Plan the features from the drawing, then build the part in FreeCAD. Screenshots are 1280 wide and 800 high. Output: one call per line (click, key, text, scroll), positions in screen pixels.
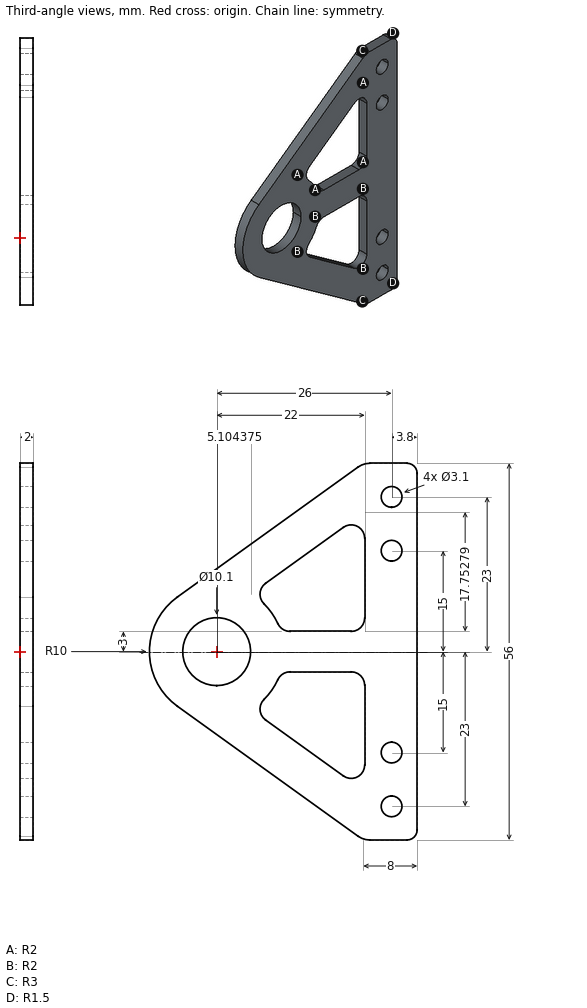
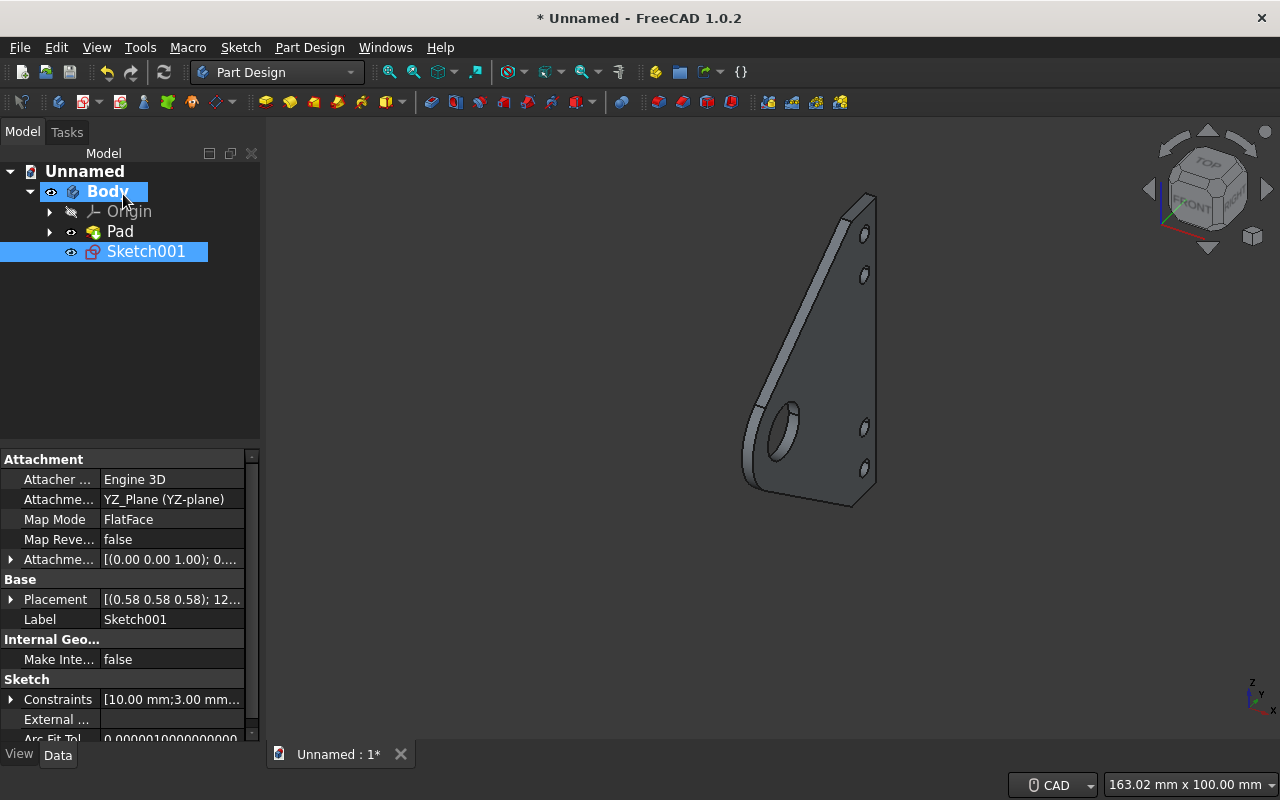
click(432, 102)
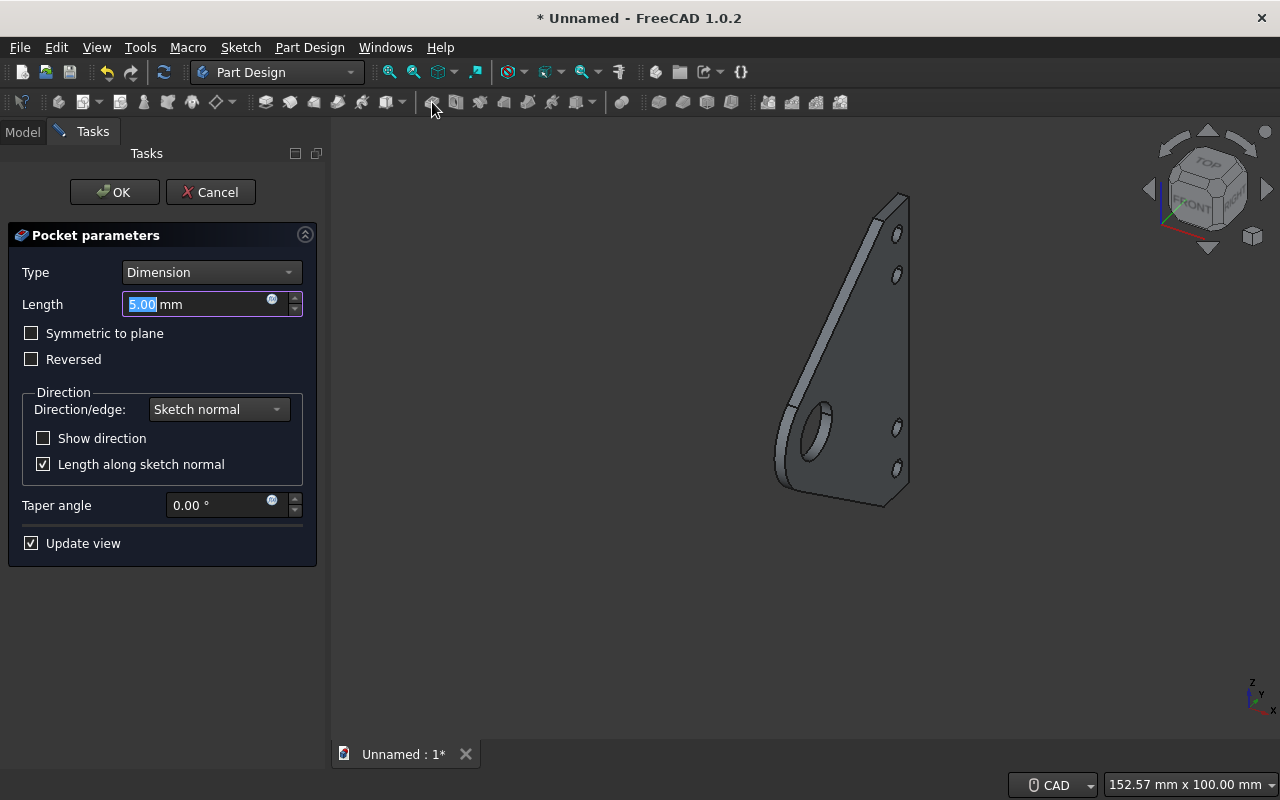
click(212, 272)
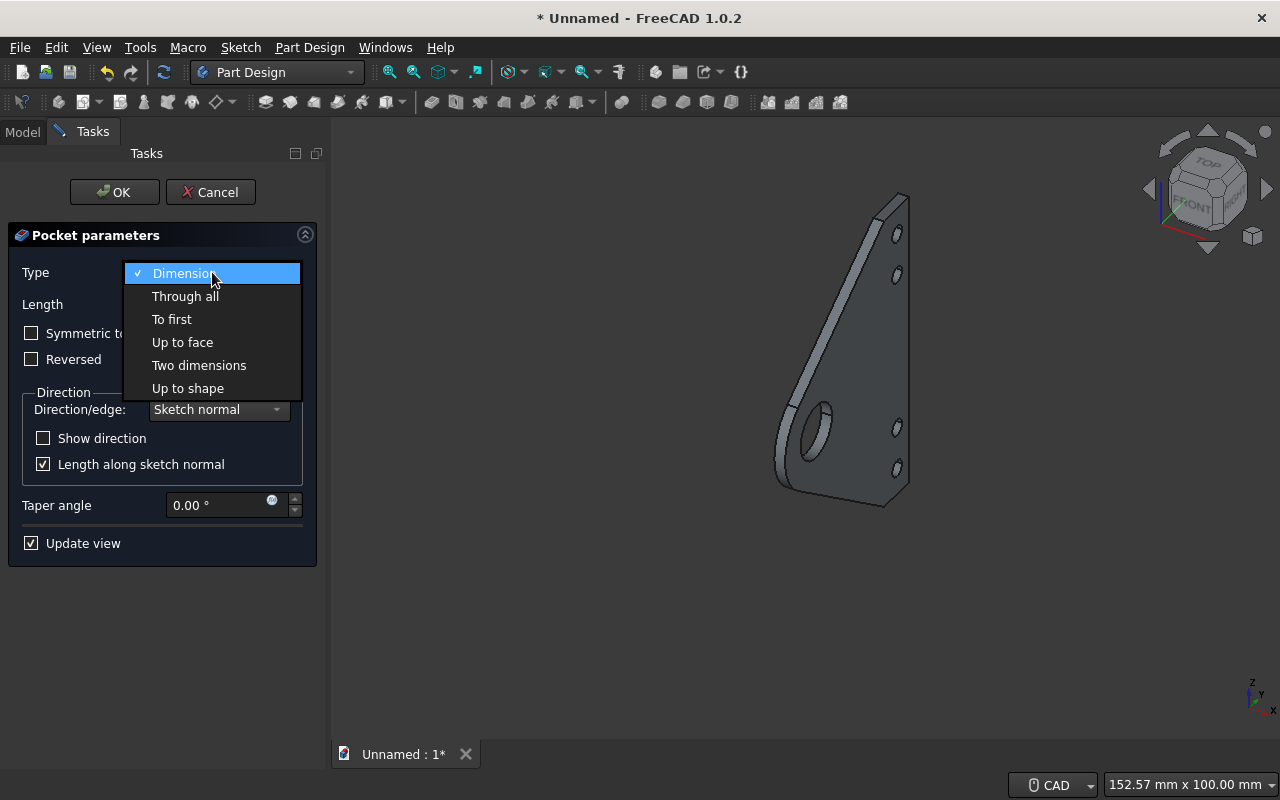
click(212, 296)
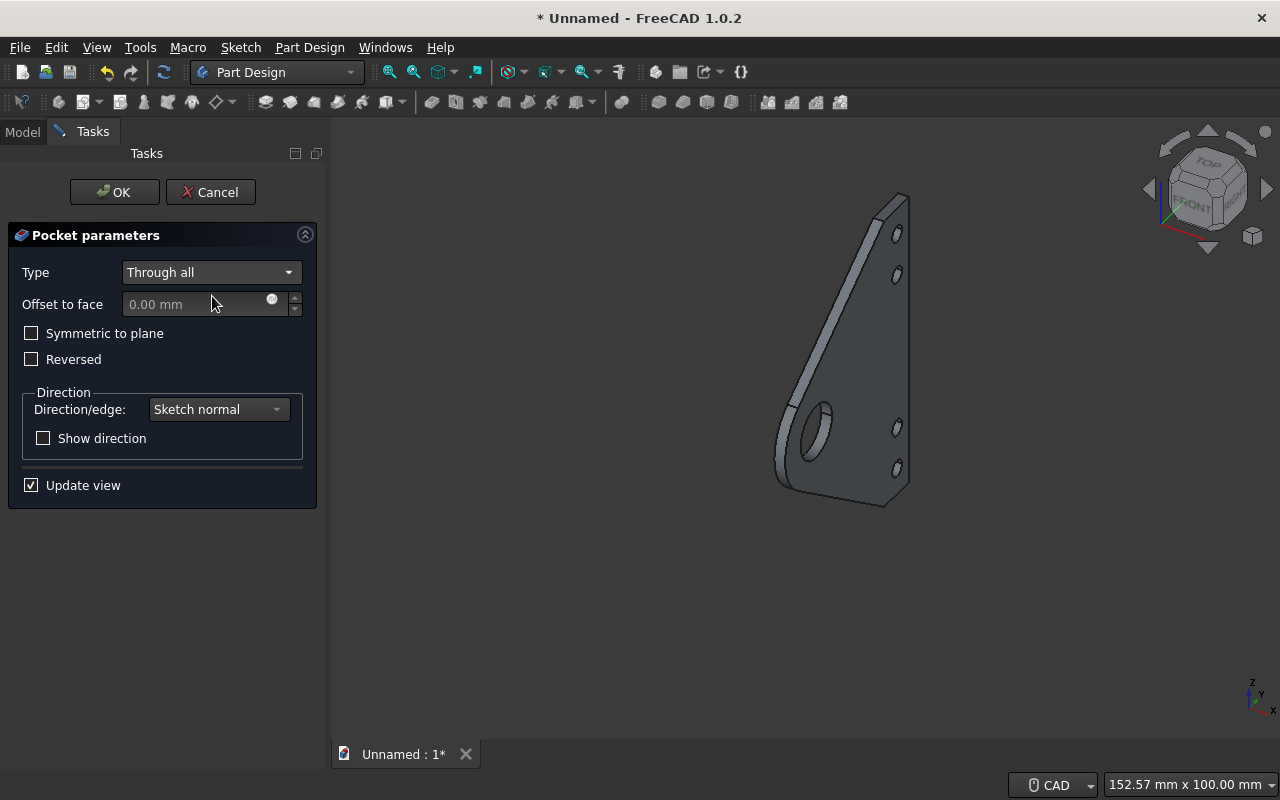
click(30, 359)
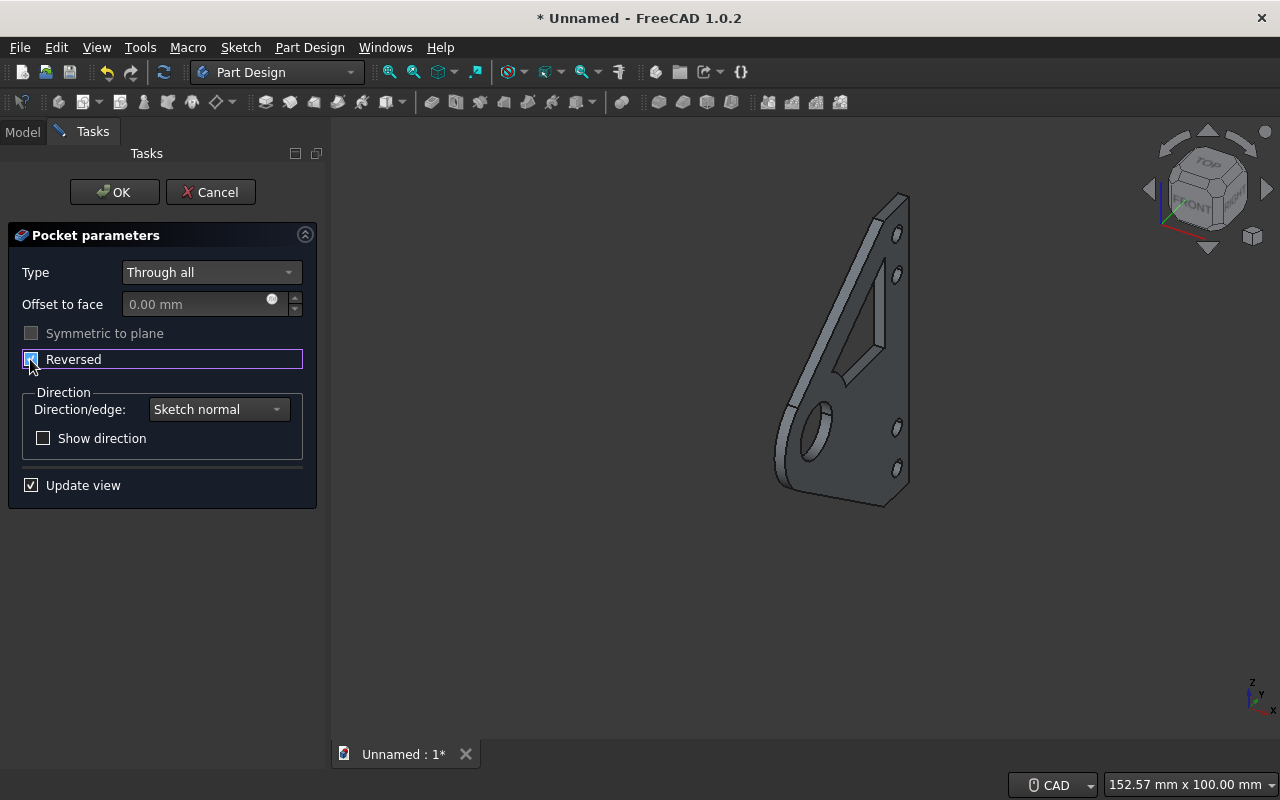
click(115, 192)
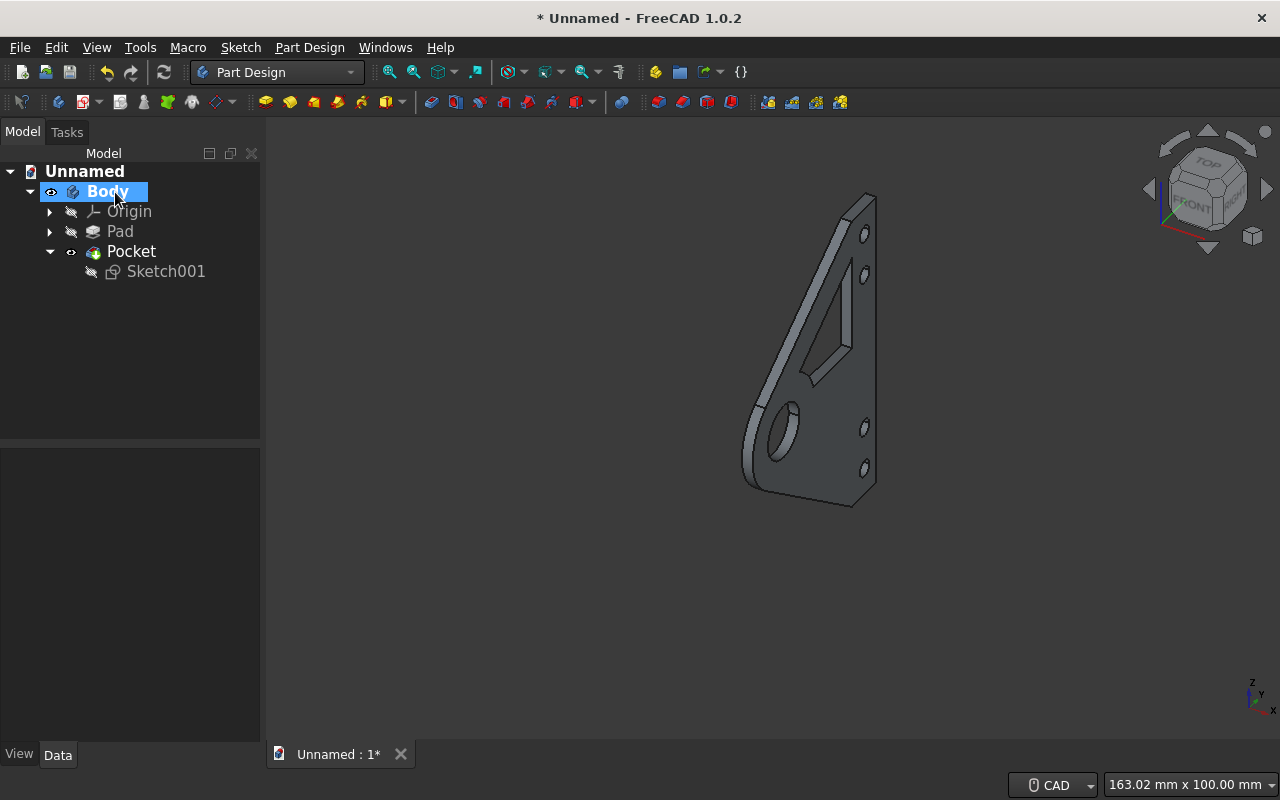
scroll(847, 346, up, 6)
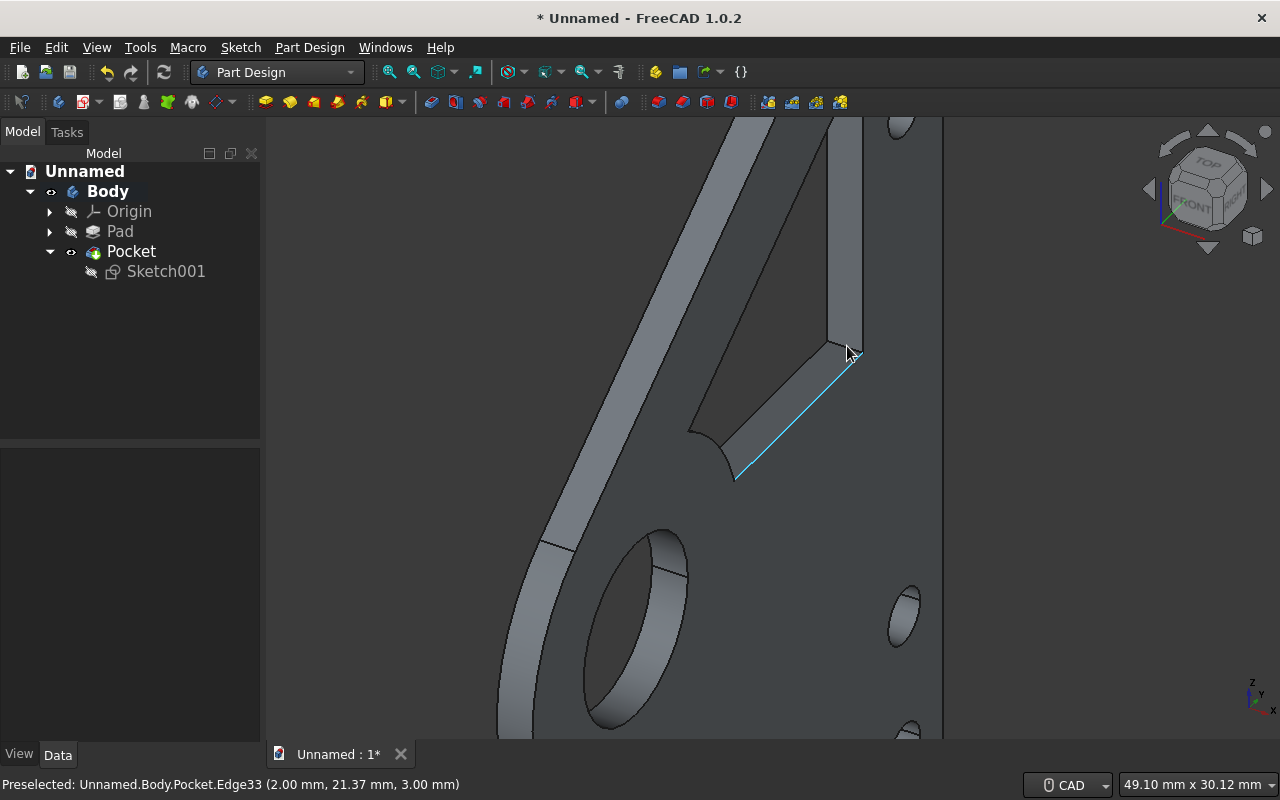
click(390, 72)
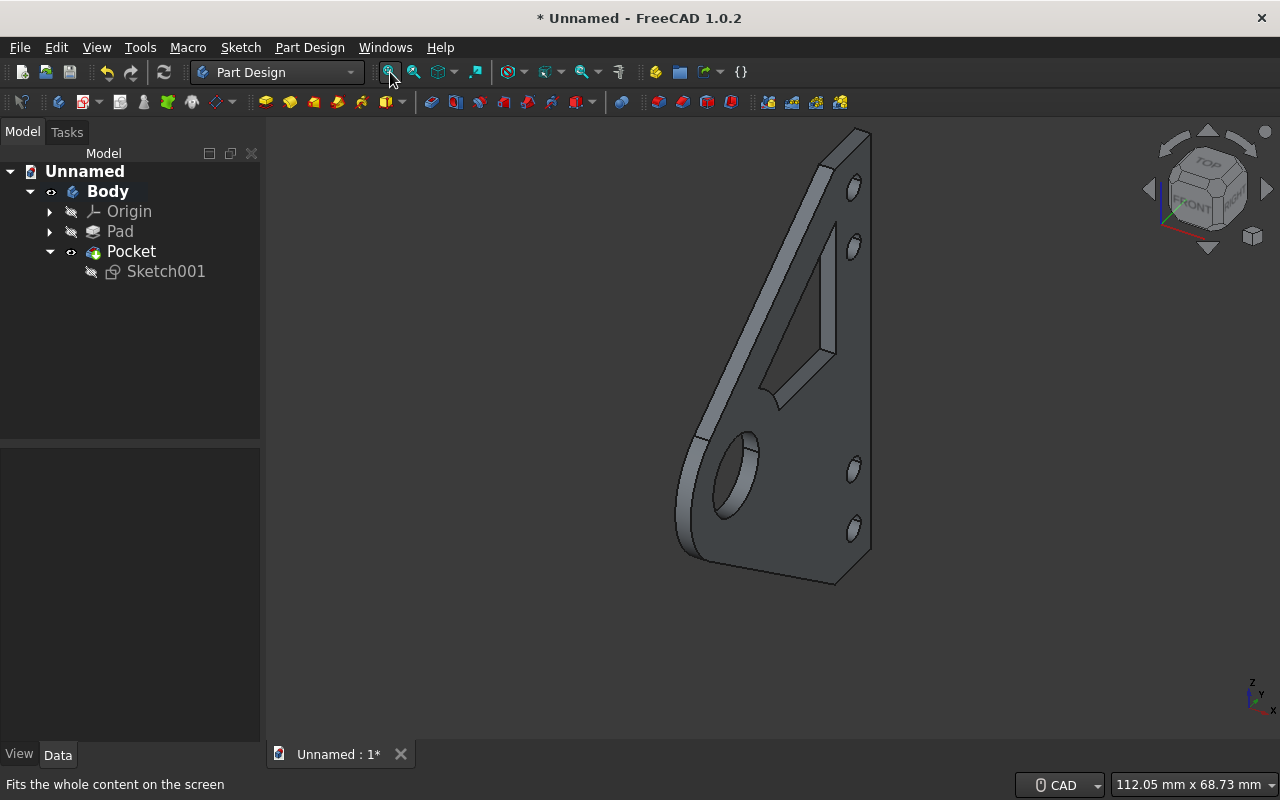
key(0)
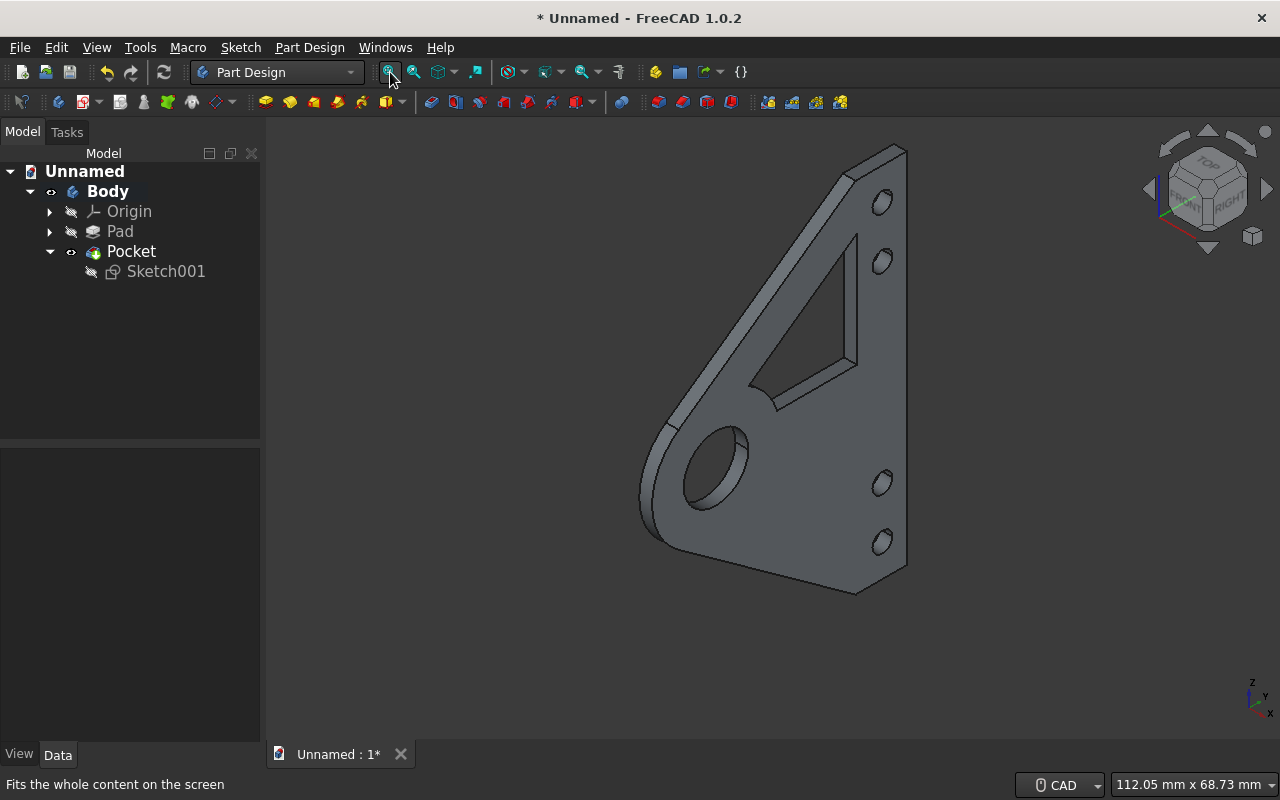
scroll(850, 360, up, 4)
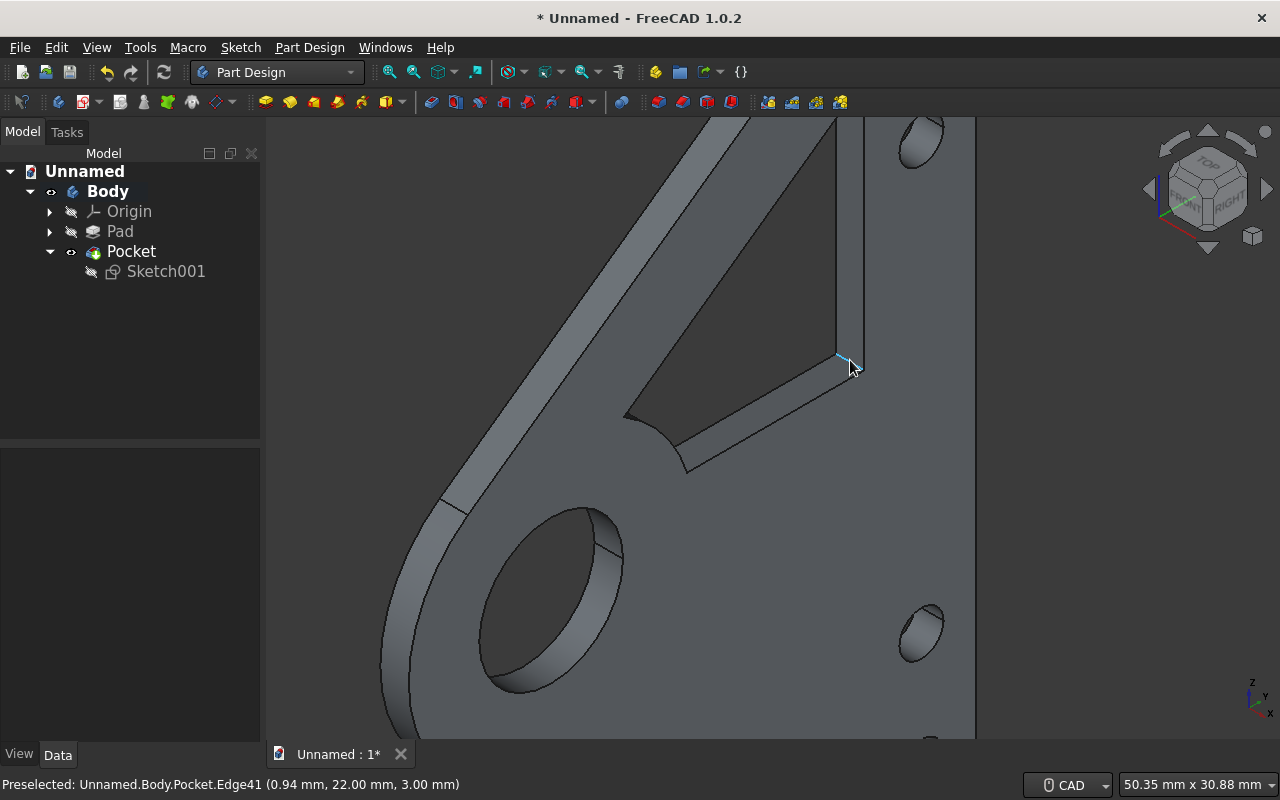
click(390, 72)